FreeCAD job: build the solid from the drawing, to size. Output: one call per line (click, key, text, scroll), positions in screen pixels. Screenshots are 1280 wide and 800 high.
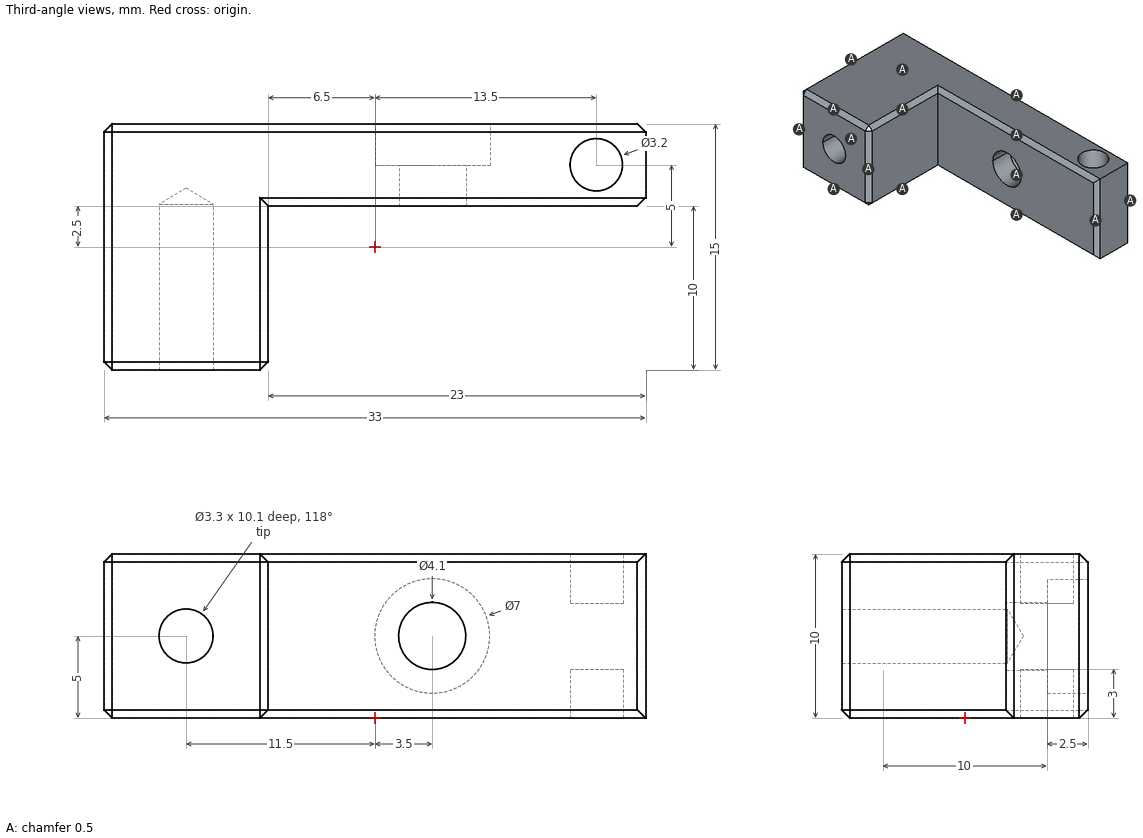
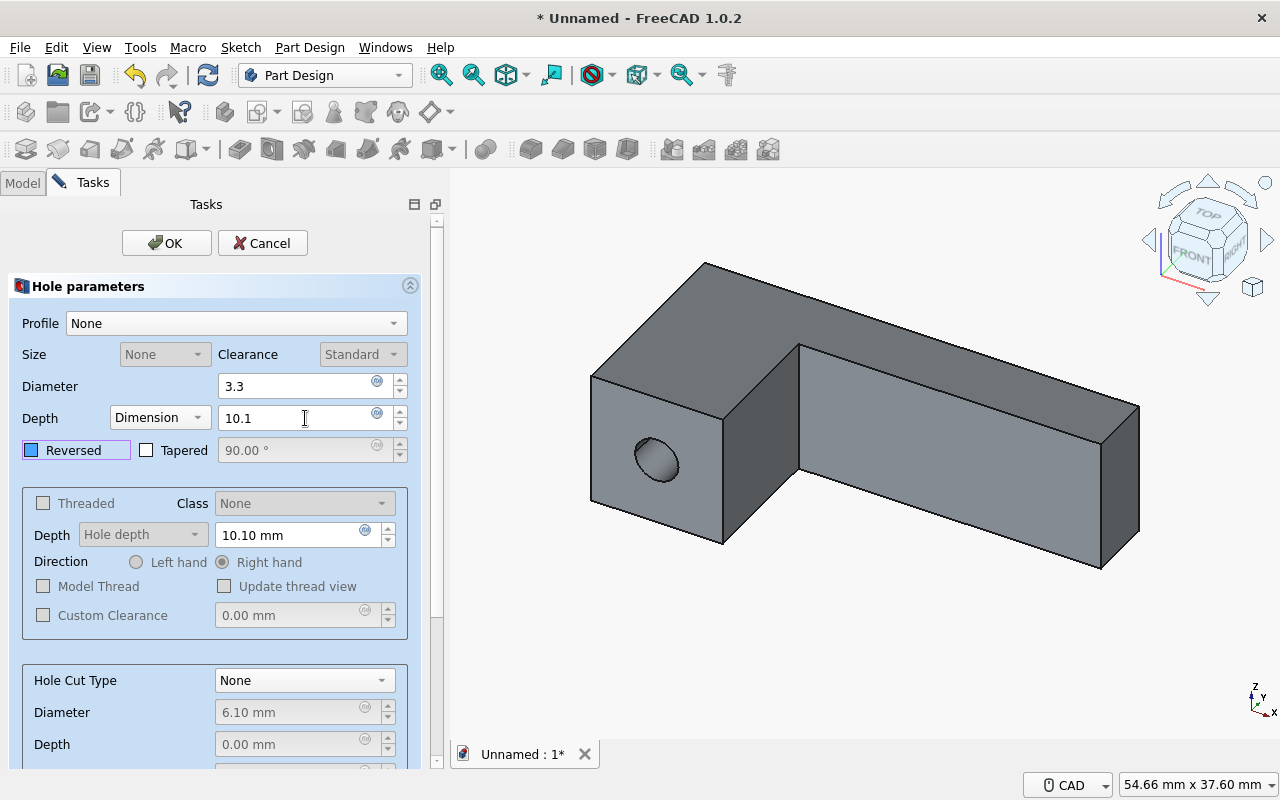
click(167, 243)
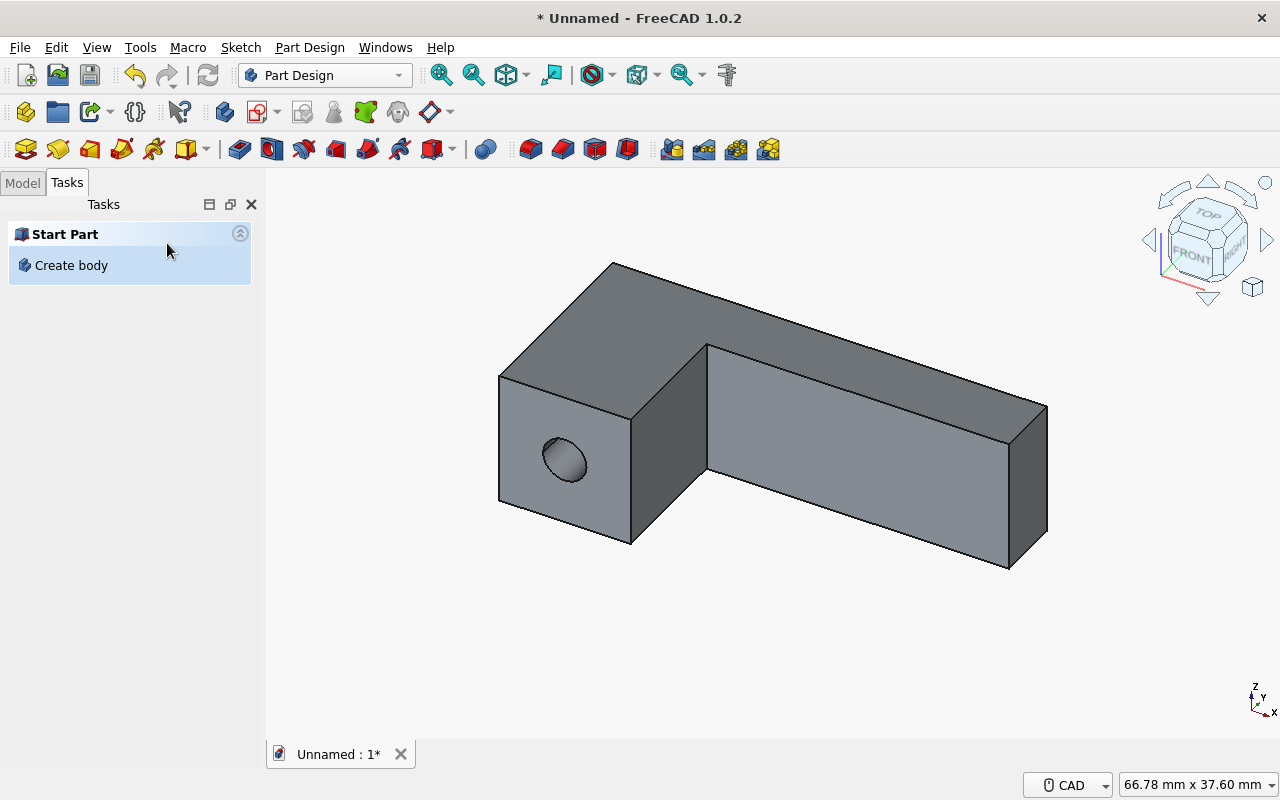
click(565, 397)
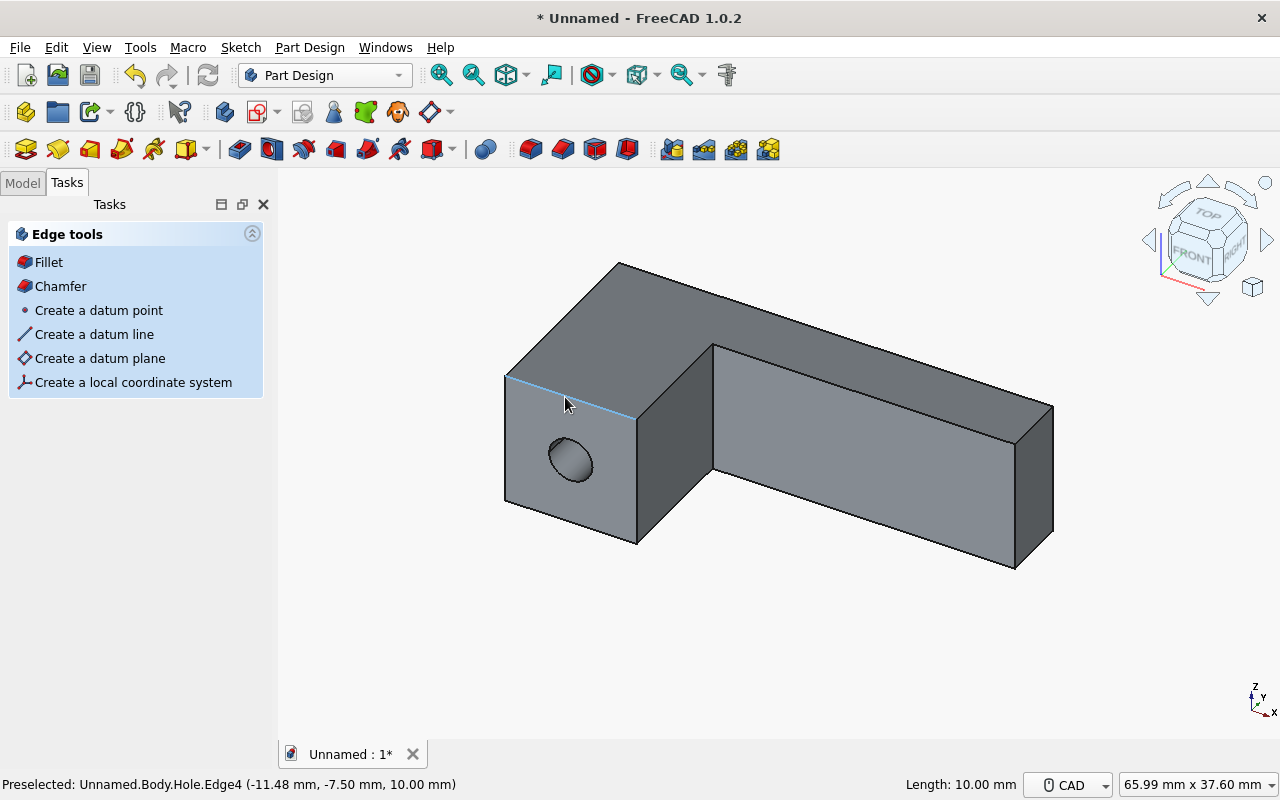
click(1015, 505, ctrl)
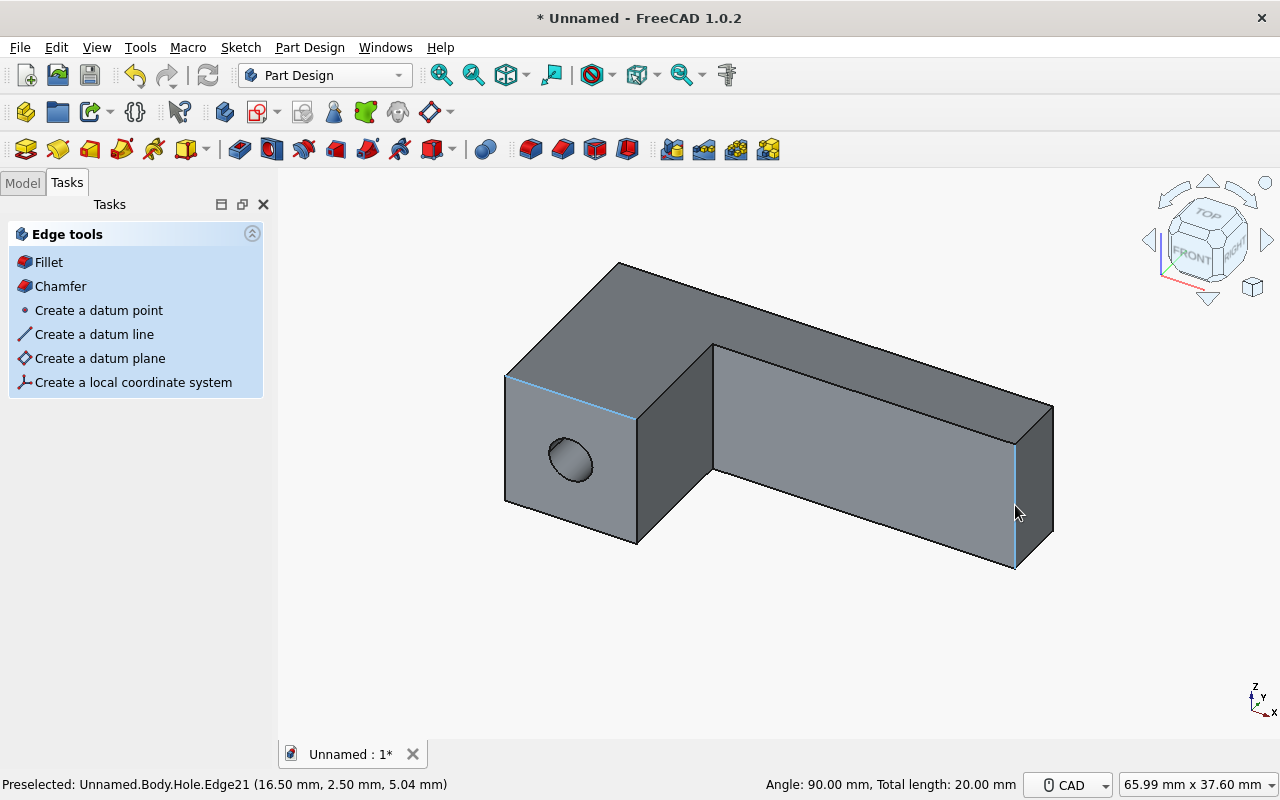
click(637, 481, ctrl)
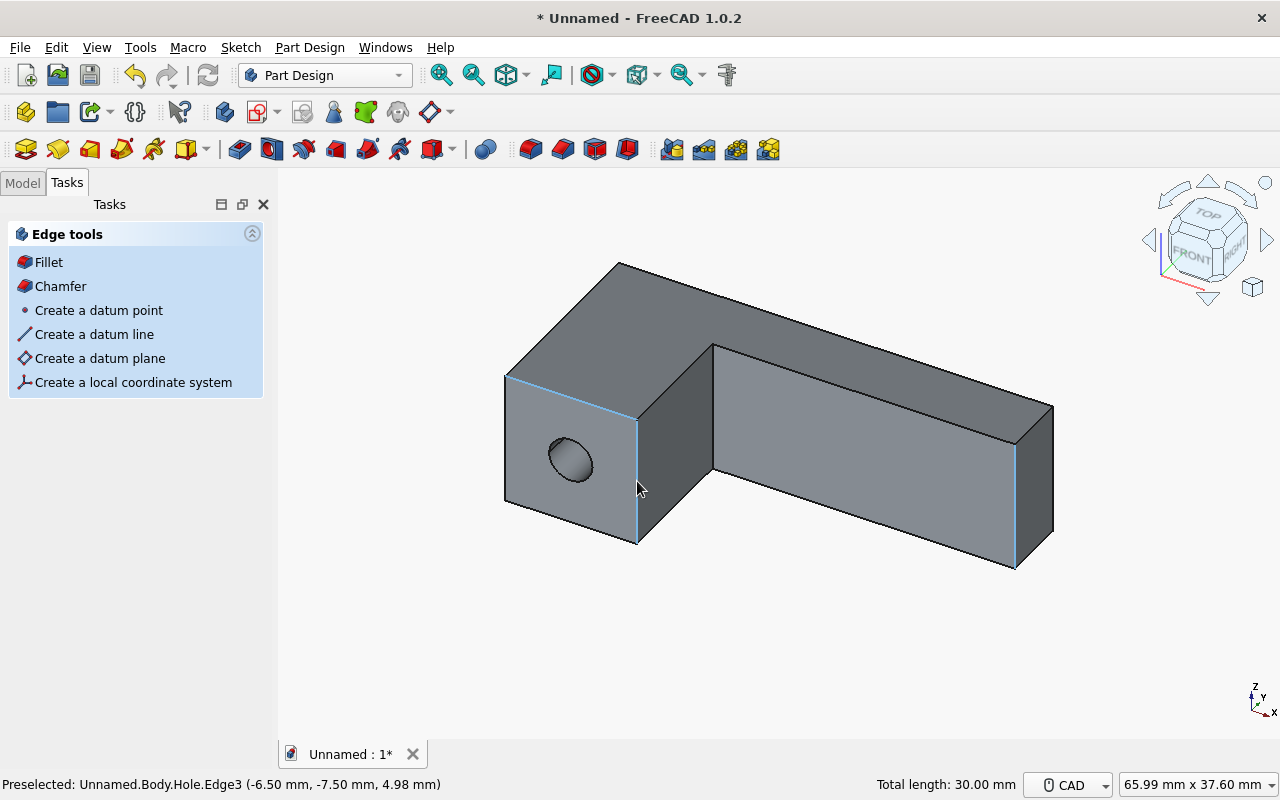
click(864, 393, ctrl)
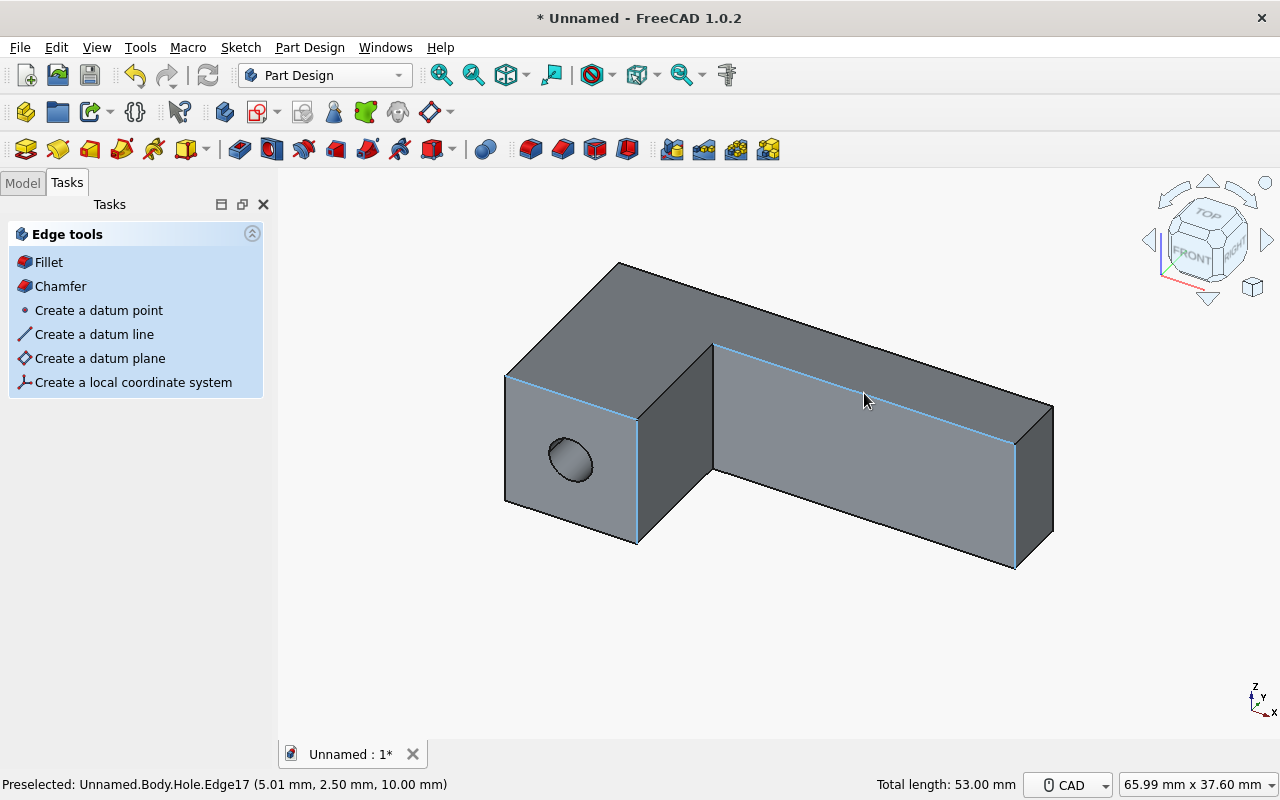
click(675, 381, ctrl)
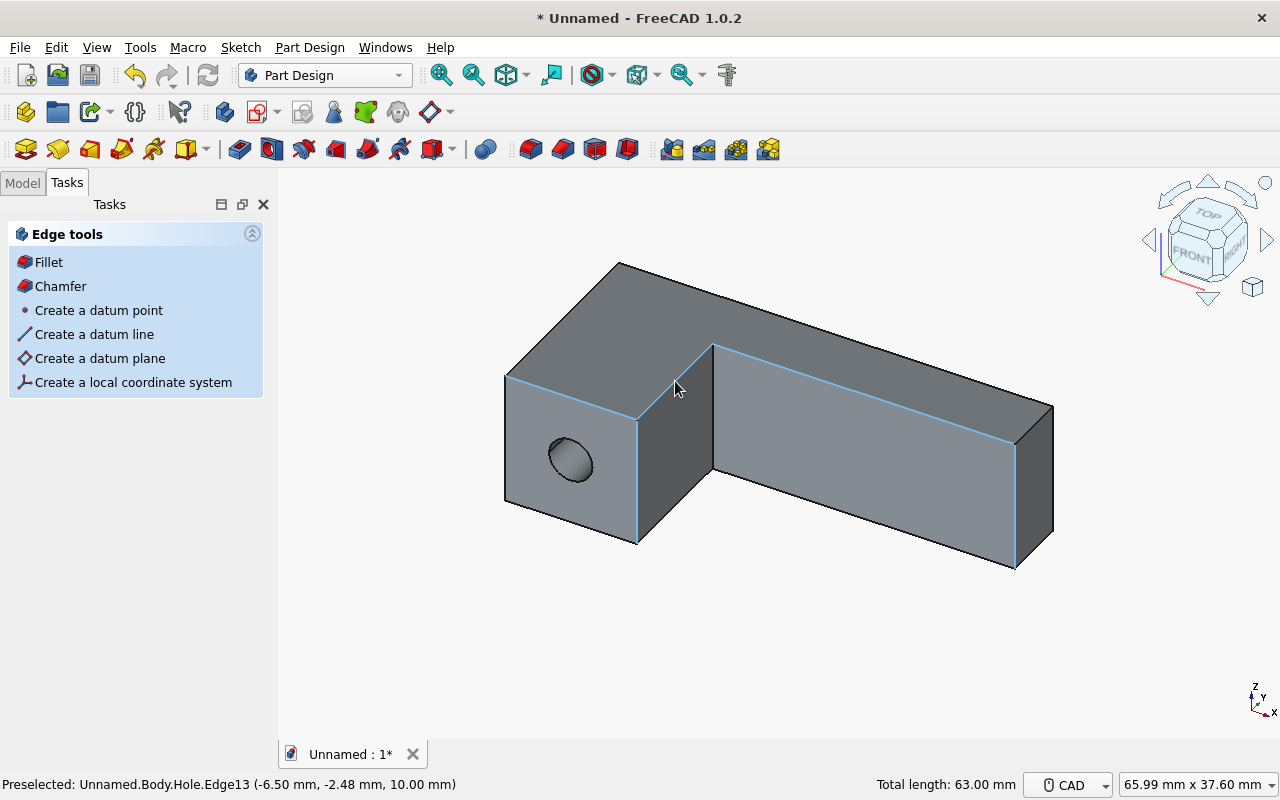
key(0)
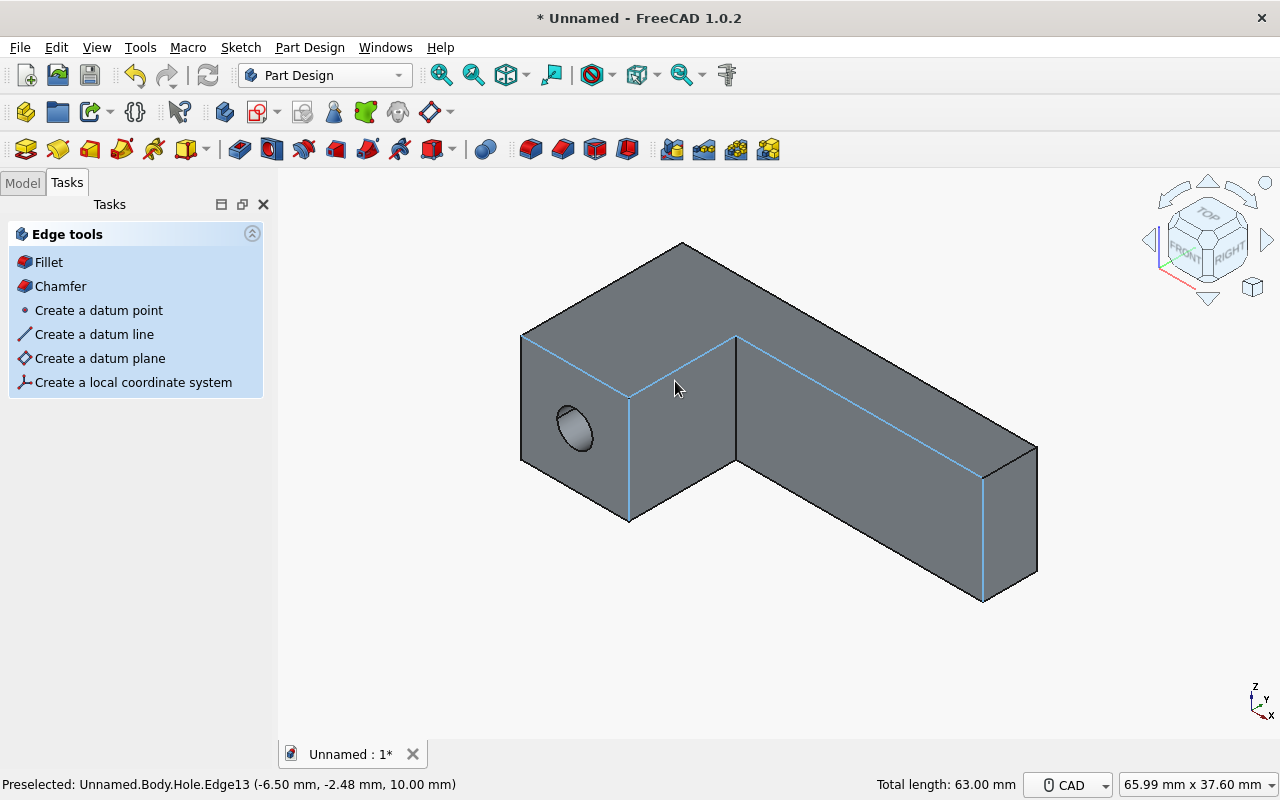
key(2)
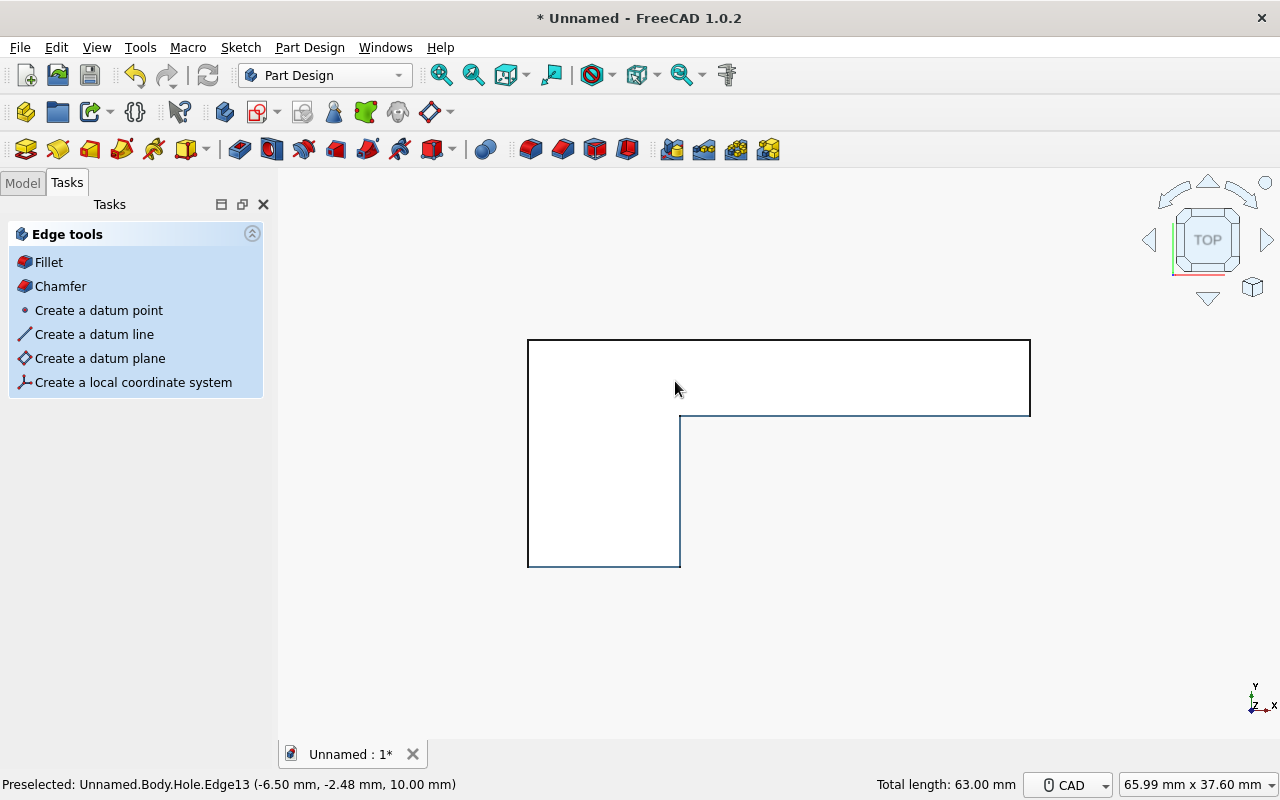
key(1)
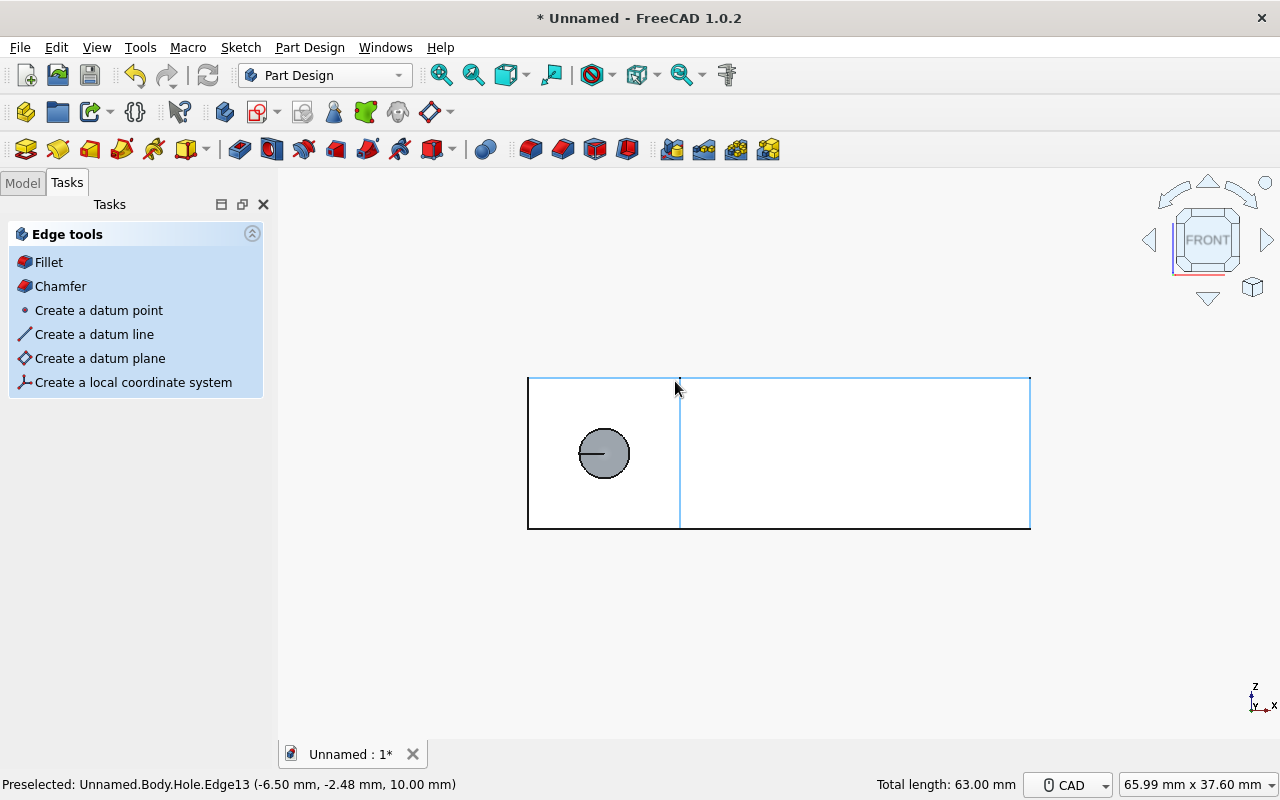
click(855, 528, ctrl)